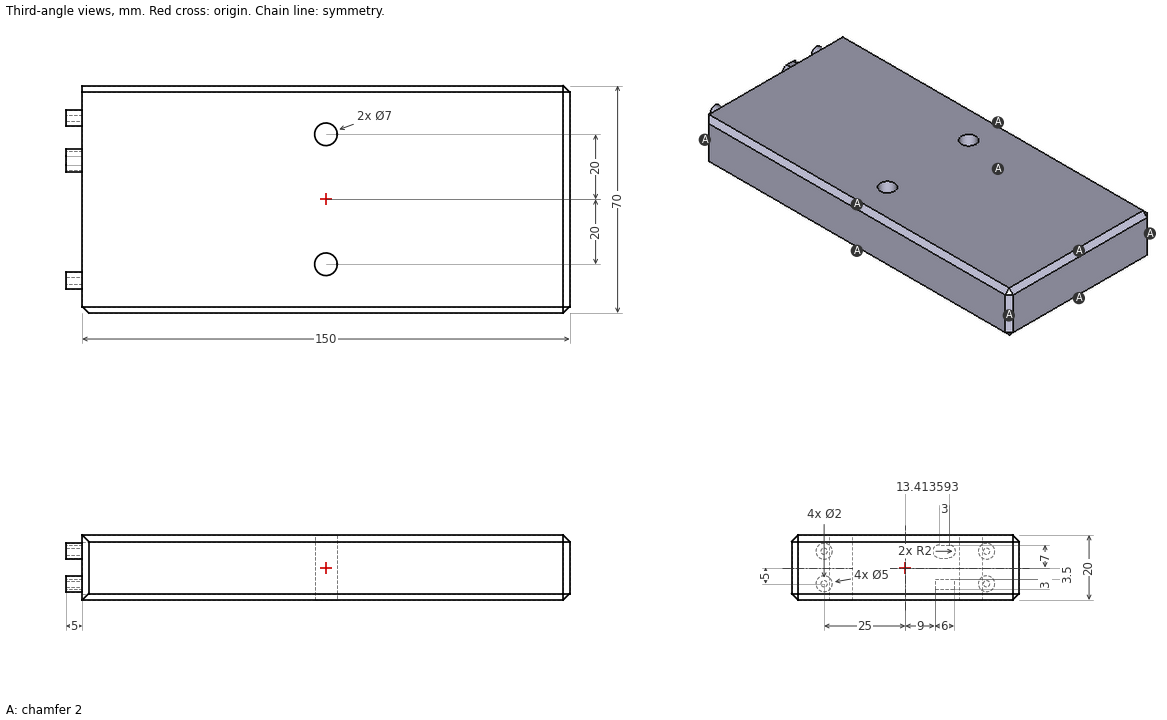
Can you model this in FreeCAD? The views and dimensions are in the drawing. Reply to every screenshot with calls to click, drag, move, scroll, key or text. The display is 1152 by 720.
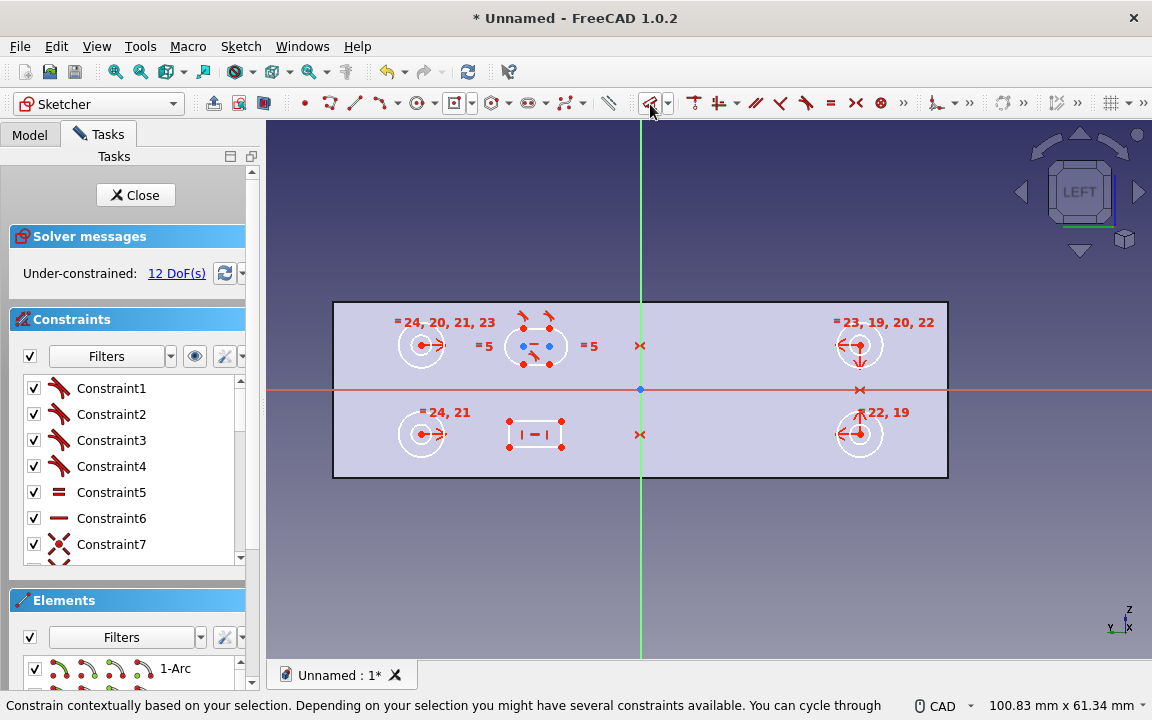
scroll(508, 336, up, 5)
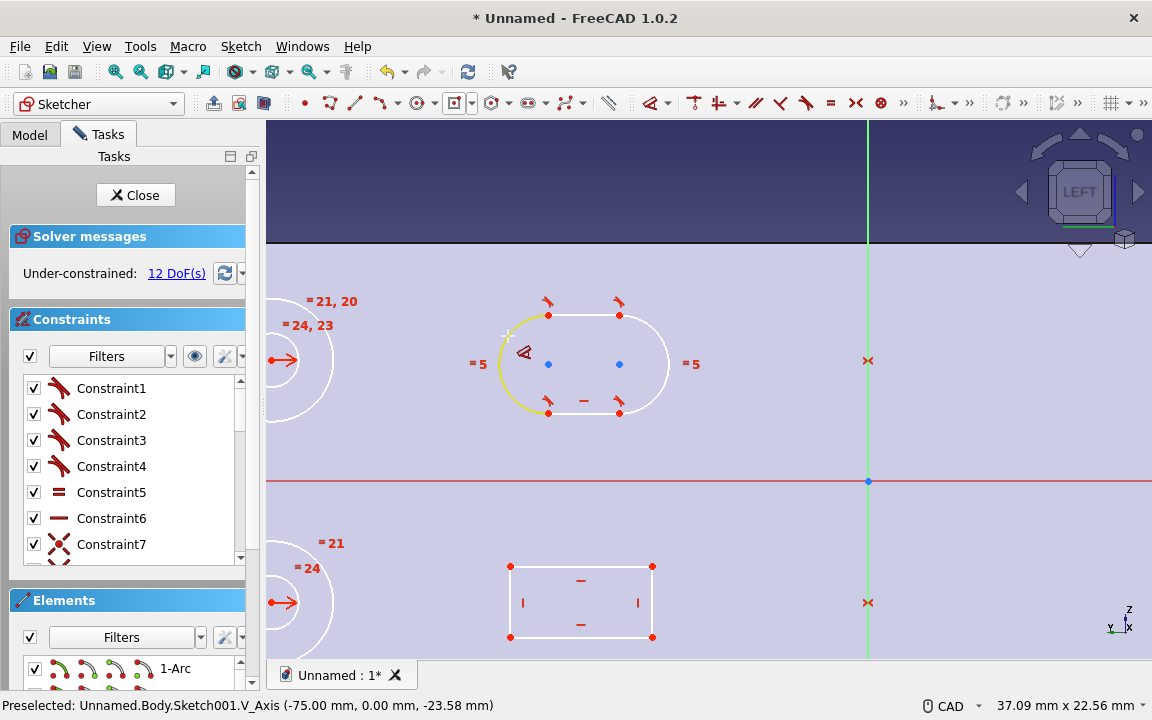
click(509, 336)
click(483, 317)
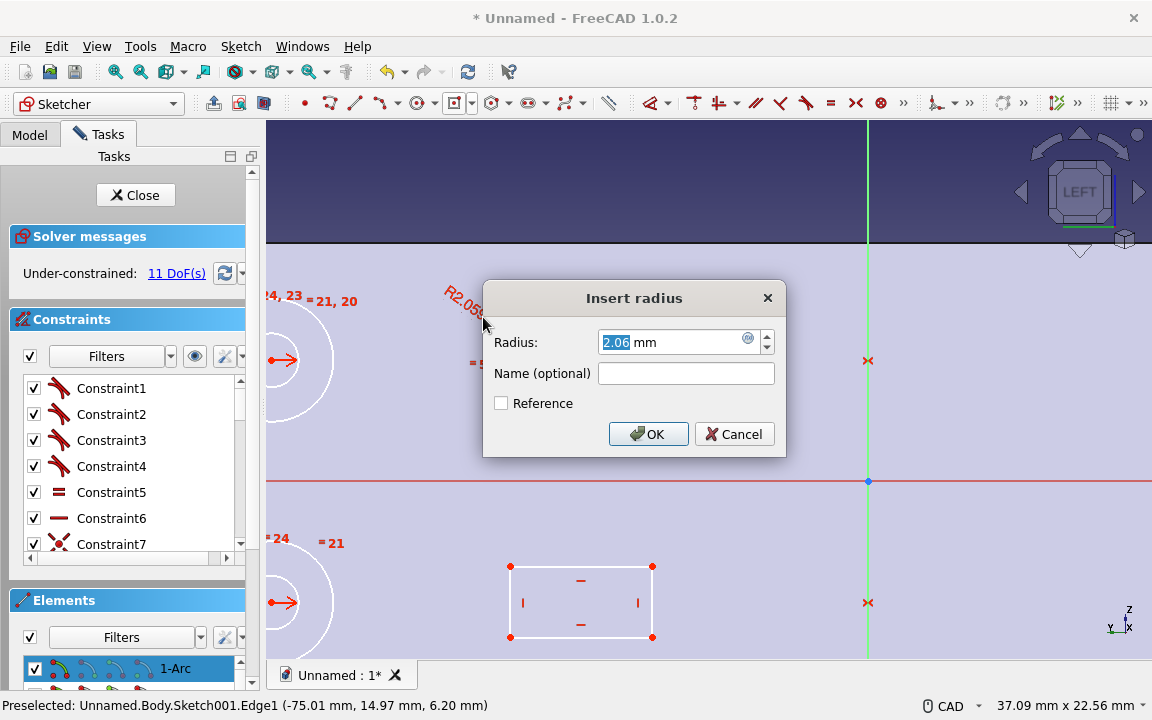
text(2)
key(Return)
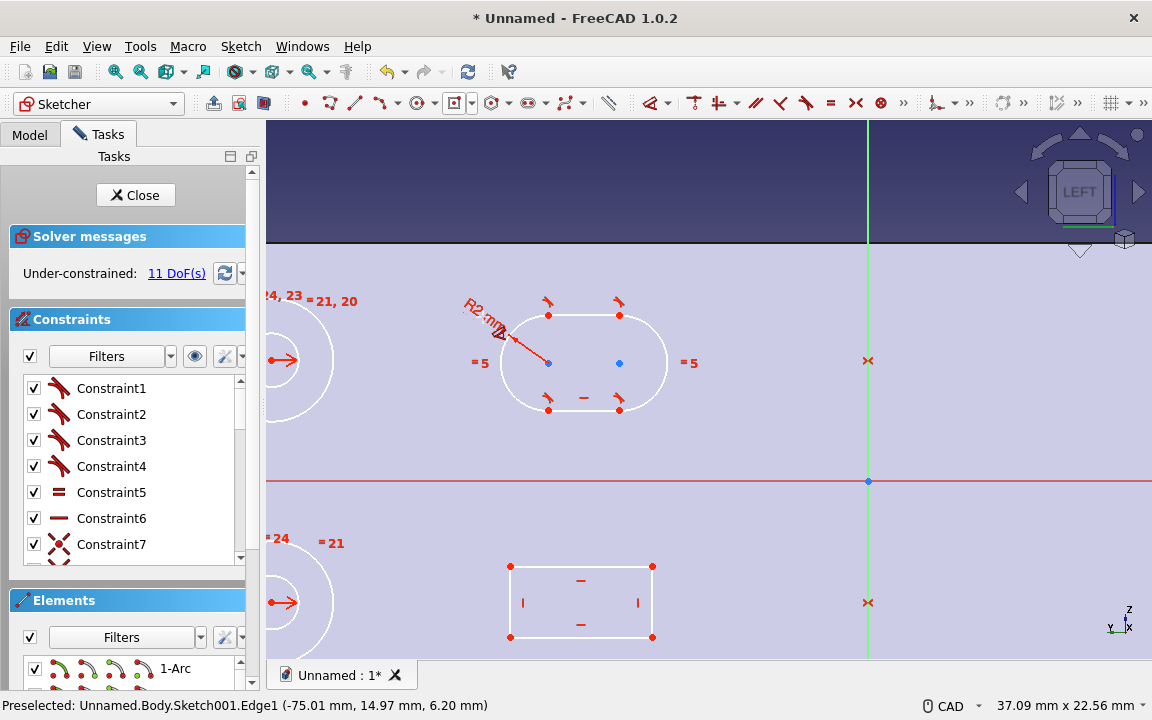
scroll(508, 336, down, 5)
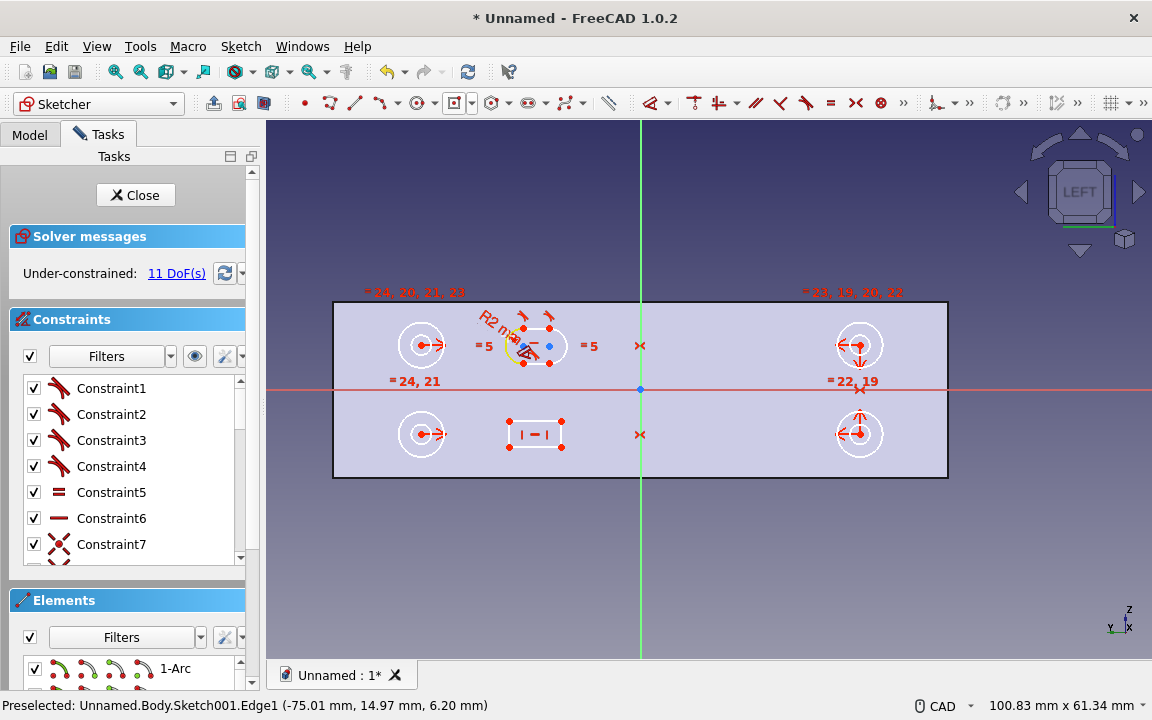
click(876, 418)
click(912, 418)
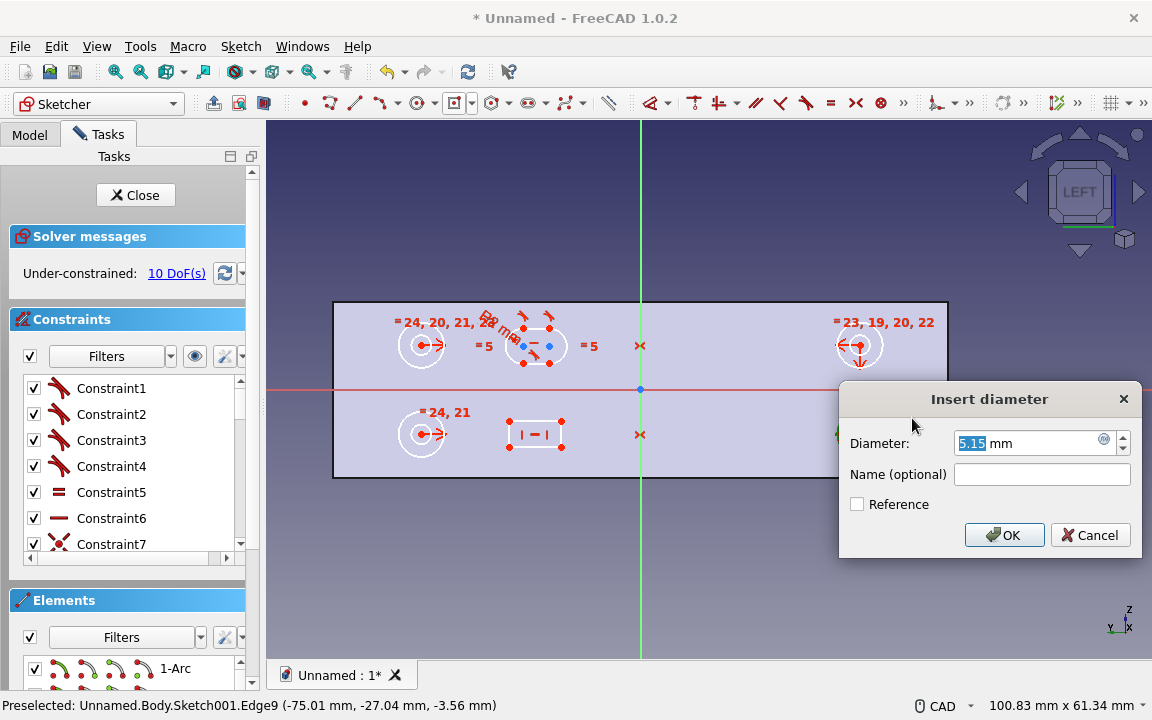
text(5)
key(Return)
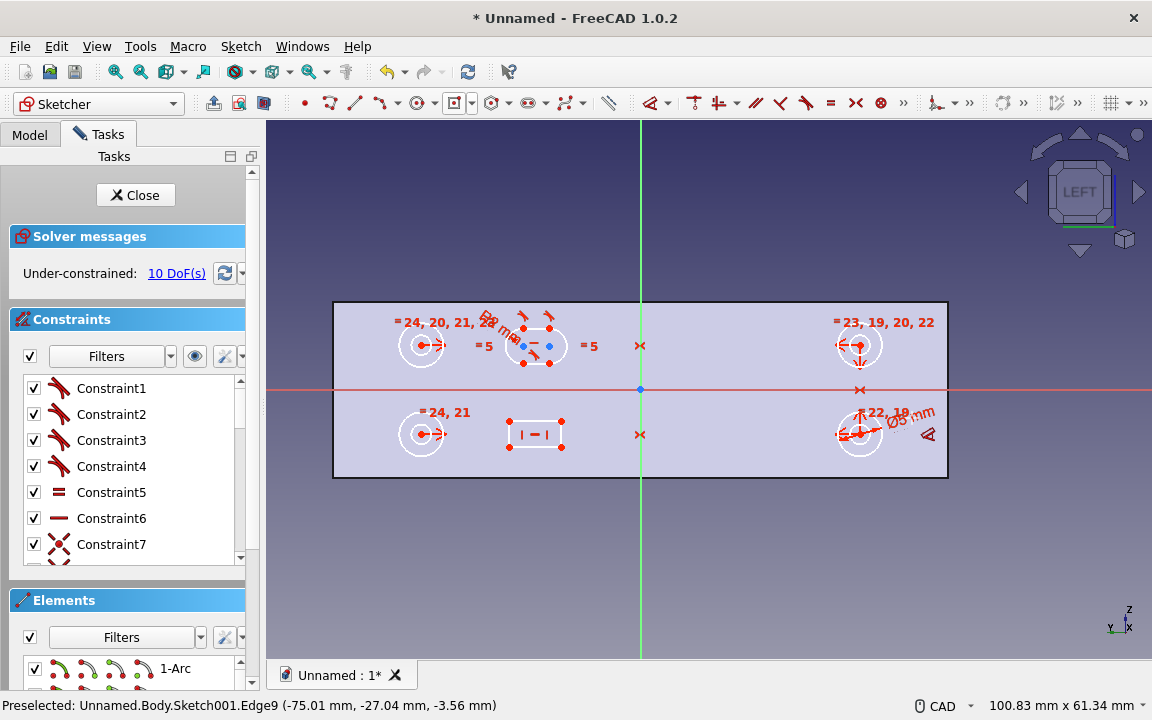
scroll(867, 427, up, 5)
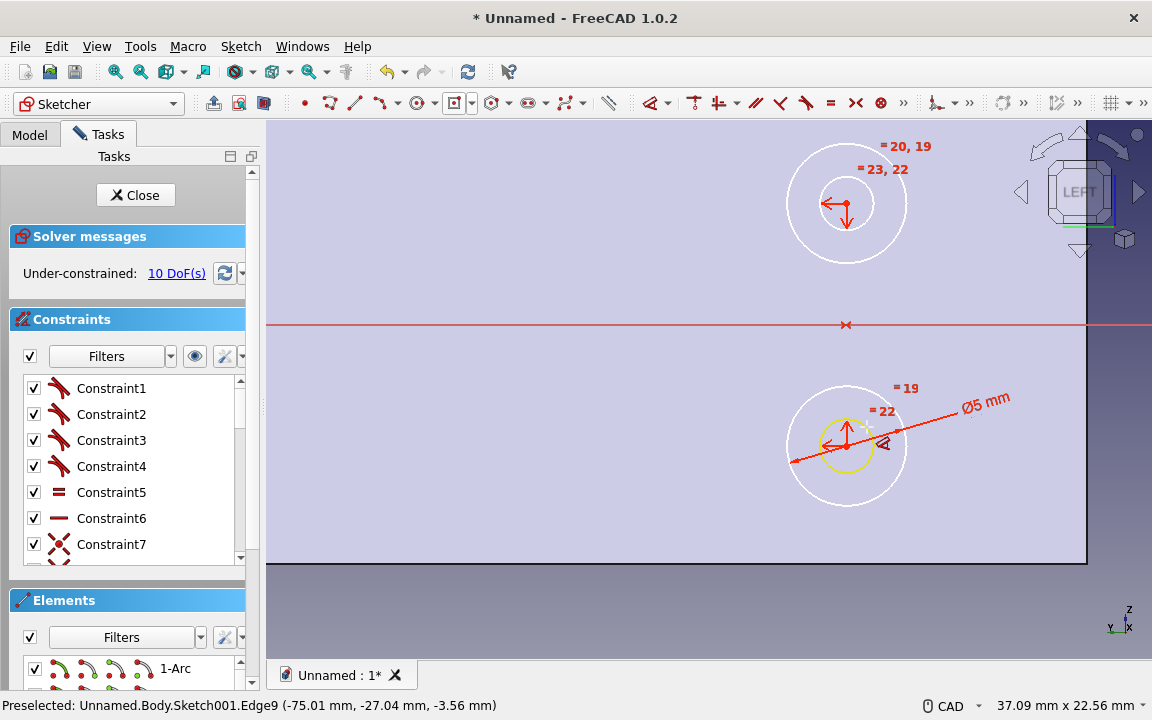
click(866, 427)
click(905, 388)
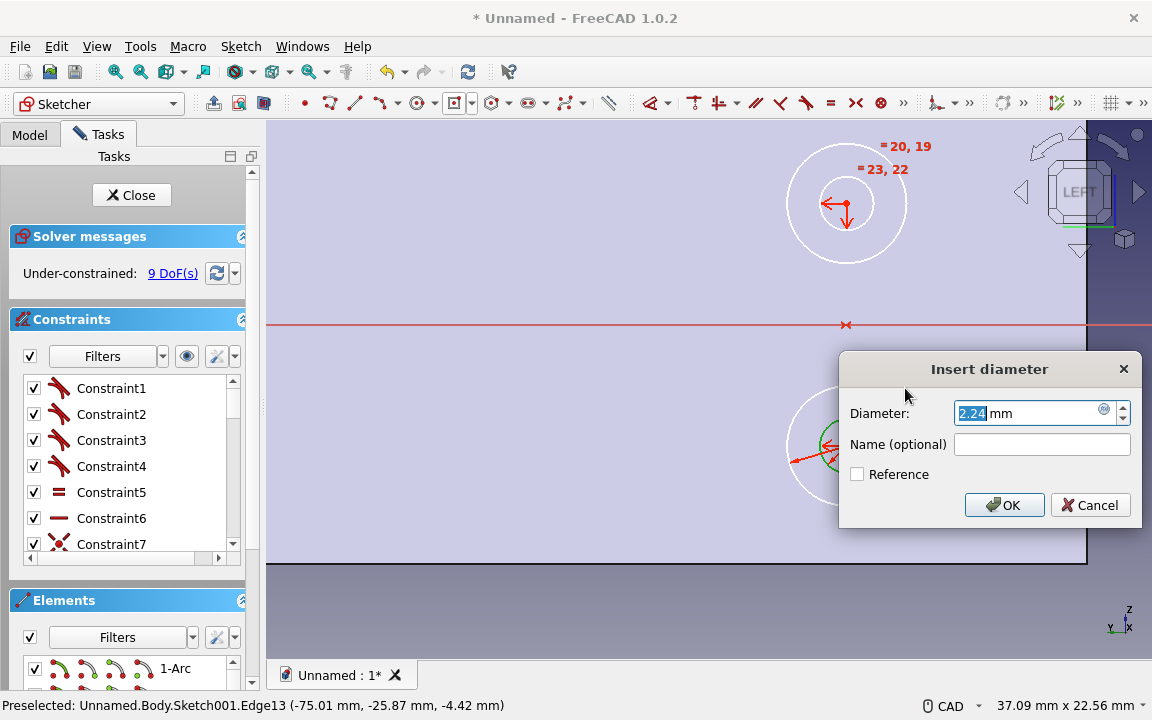
text(2)
key(Return)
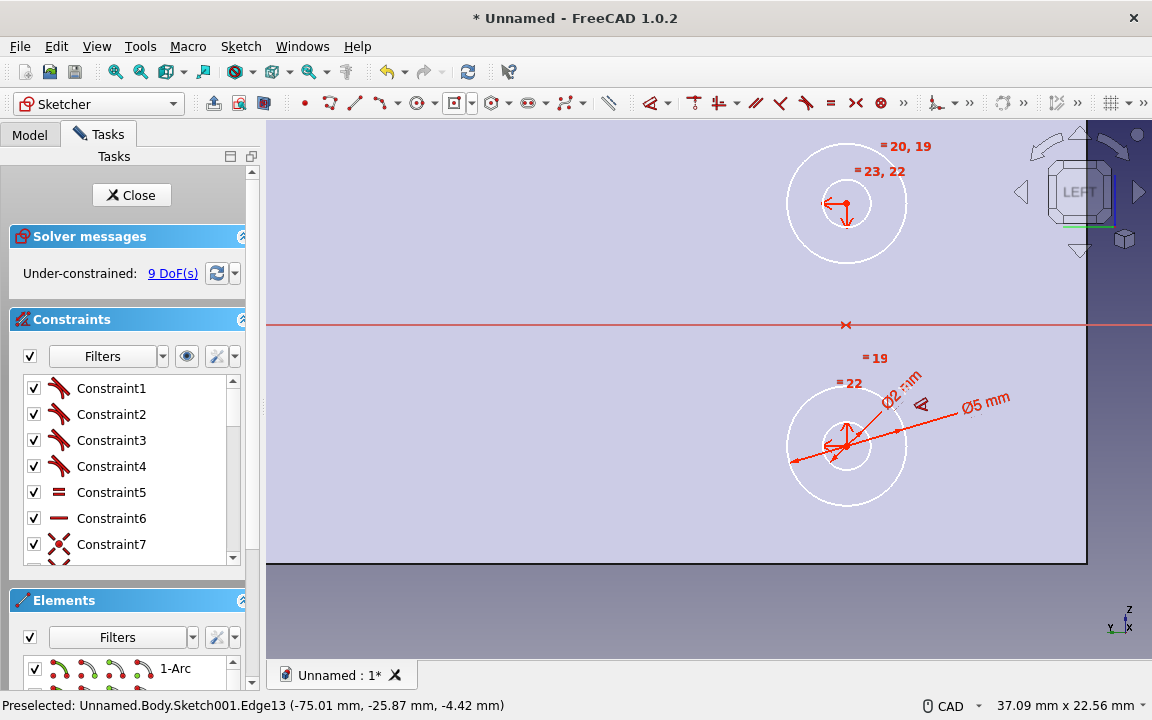
scroll(867, 427, down, 5)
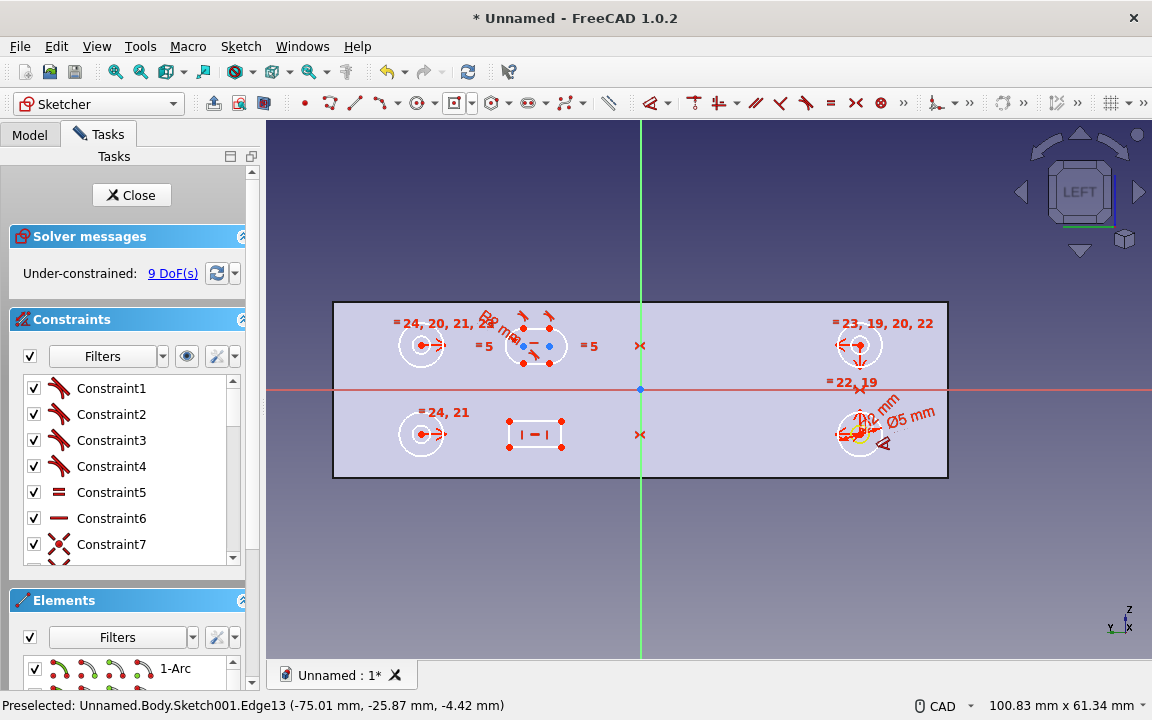
scroll(531, 329, up, 3)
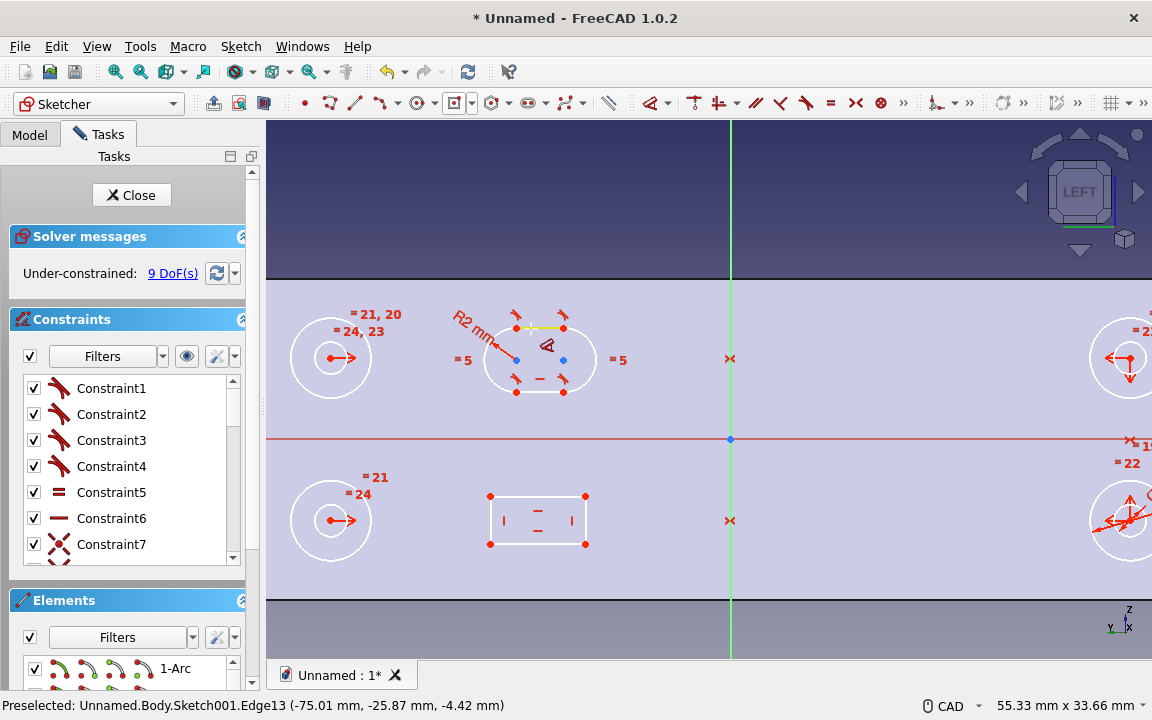
click(531, 328)
click(540, 294)